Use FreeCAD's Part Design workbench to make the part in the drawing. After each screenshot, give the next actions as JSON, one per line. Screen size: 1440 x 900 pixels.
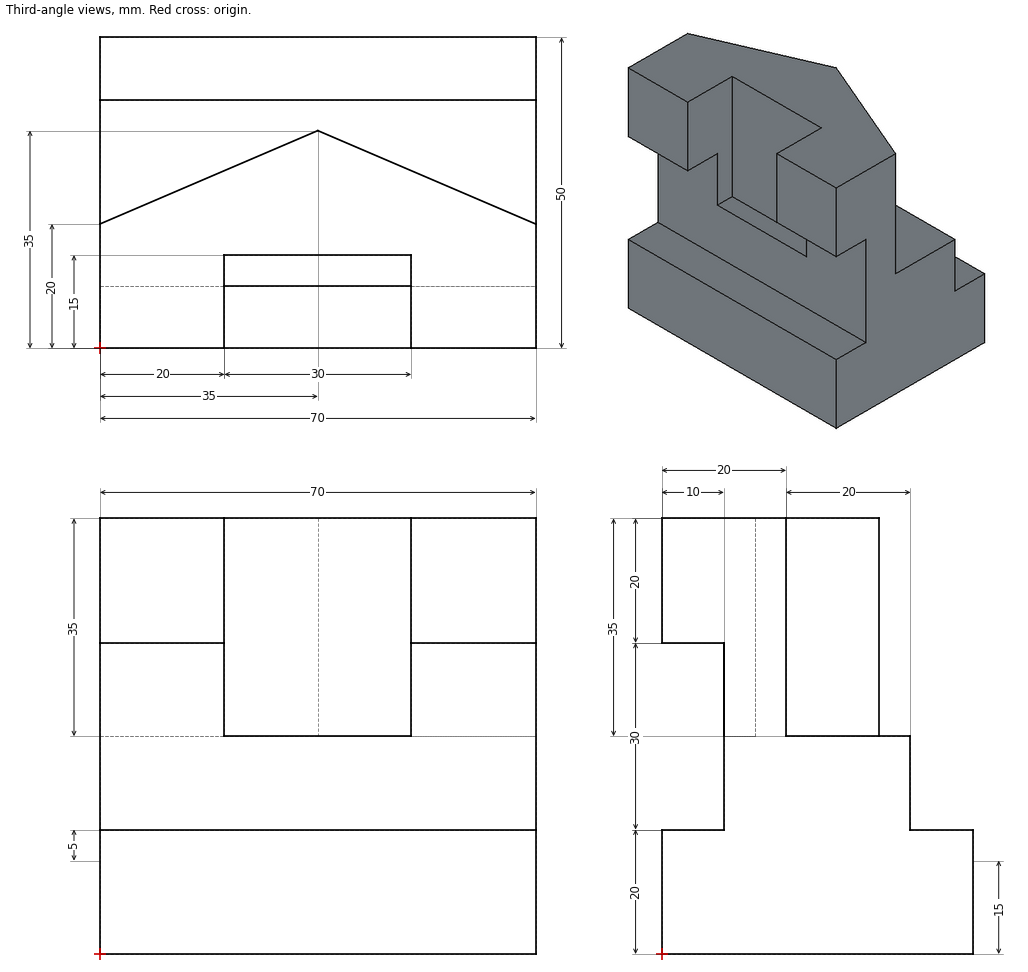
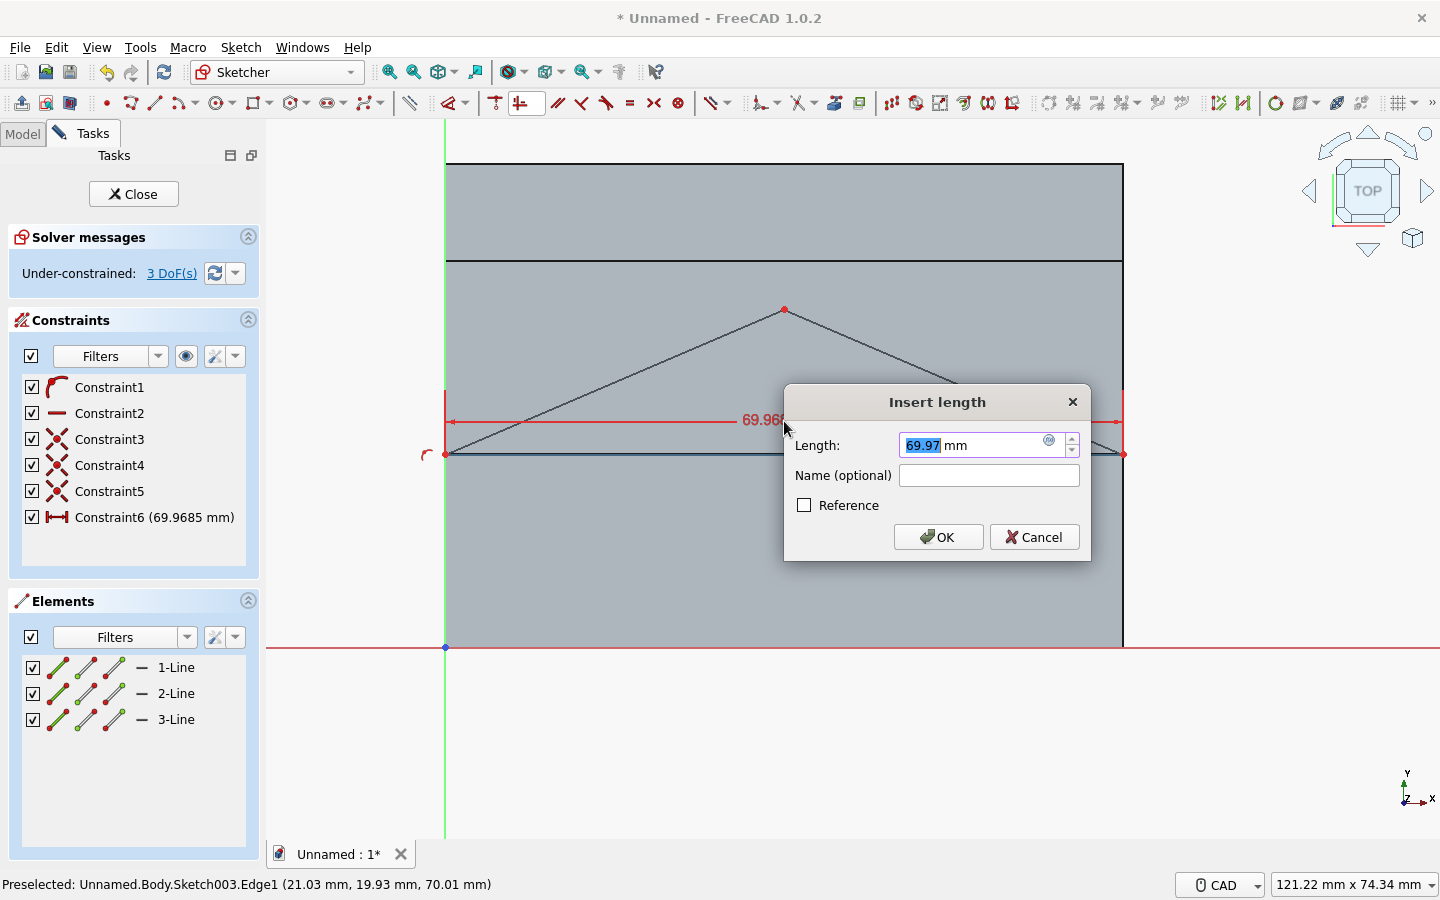
{"action": "type", "text": "70"}
{"action": "key", "text": "Return"}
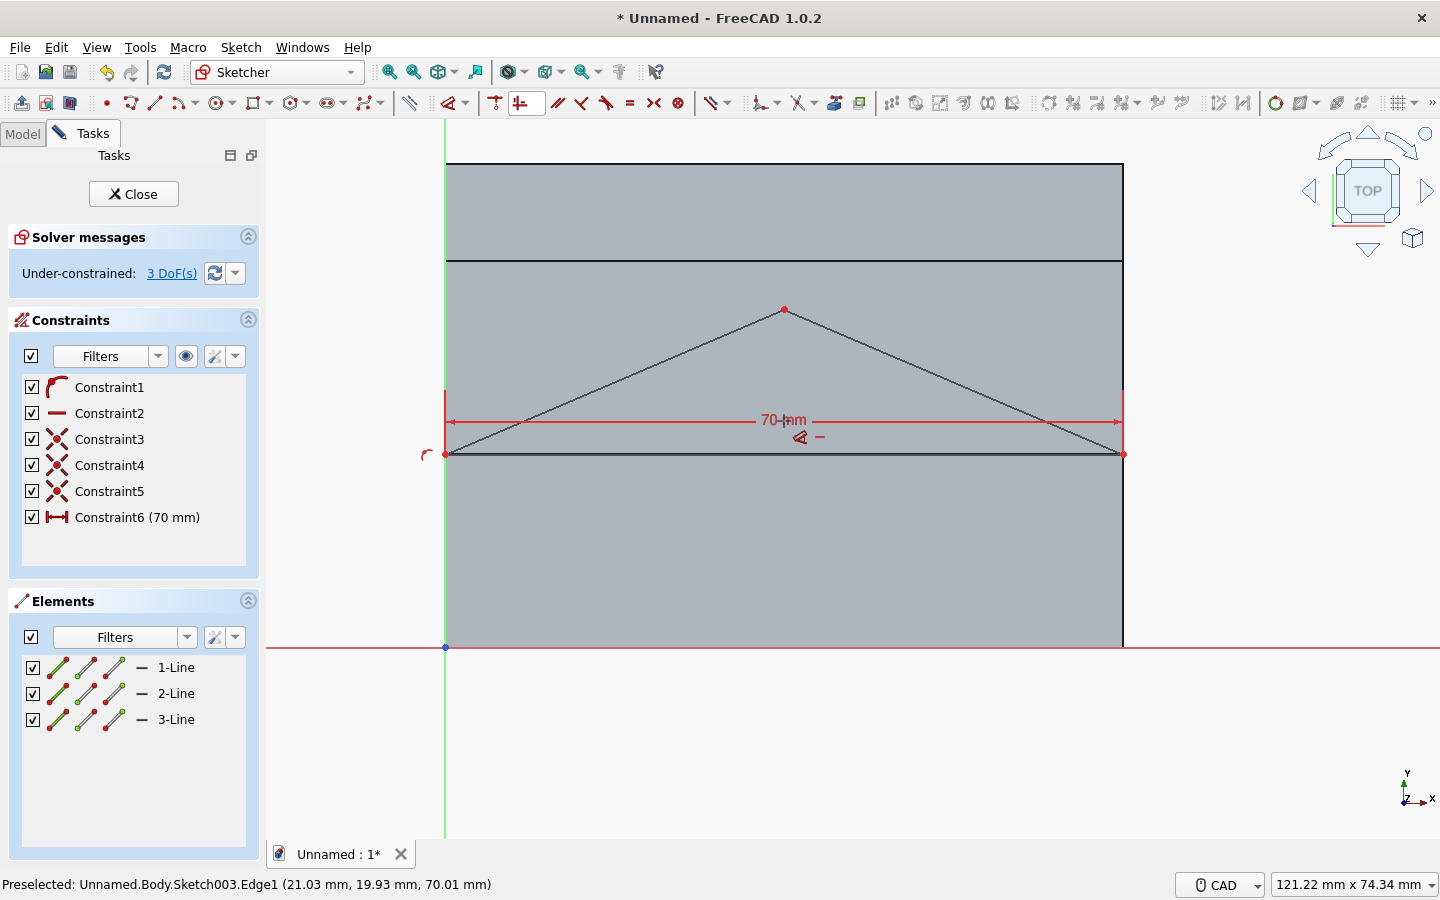
{"action": "left_click", "coordinate": [445, 455]}
{"action": "left_click", "coordinate": [411, 551]}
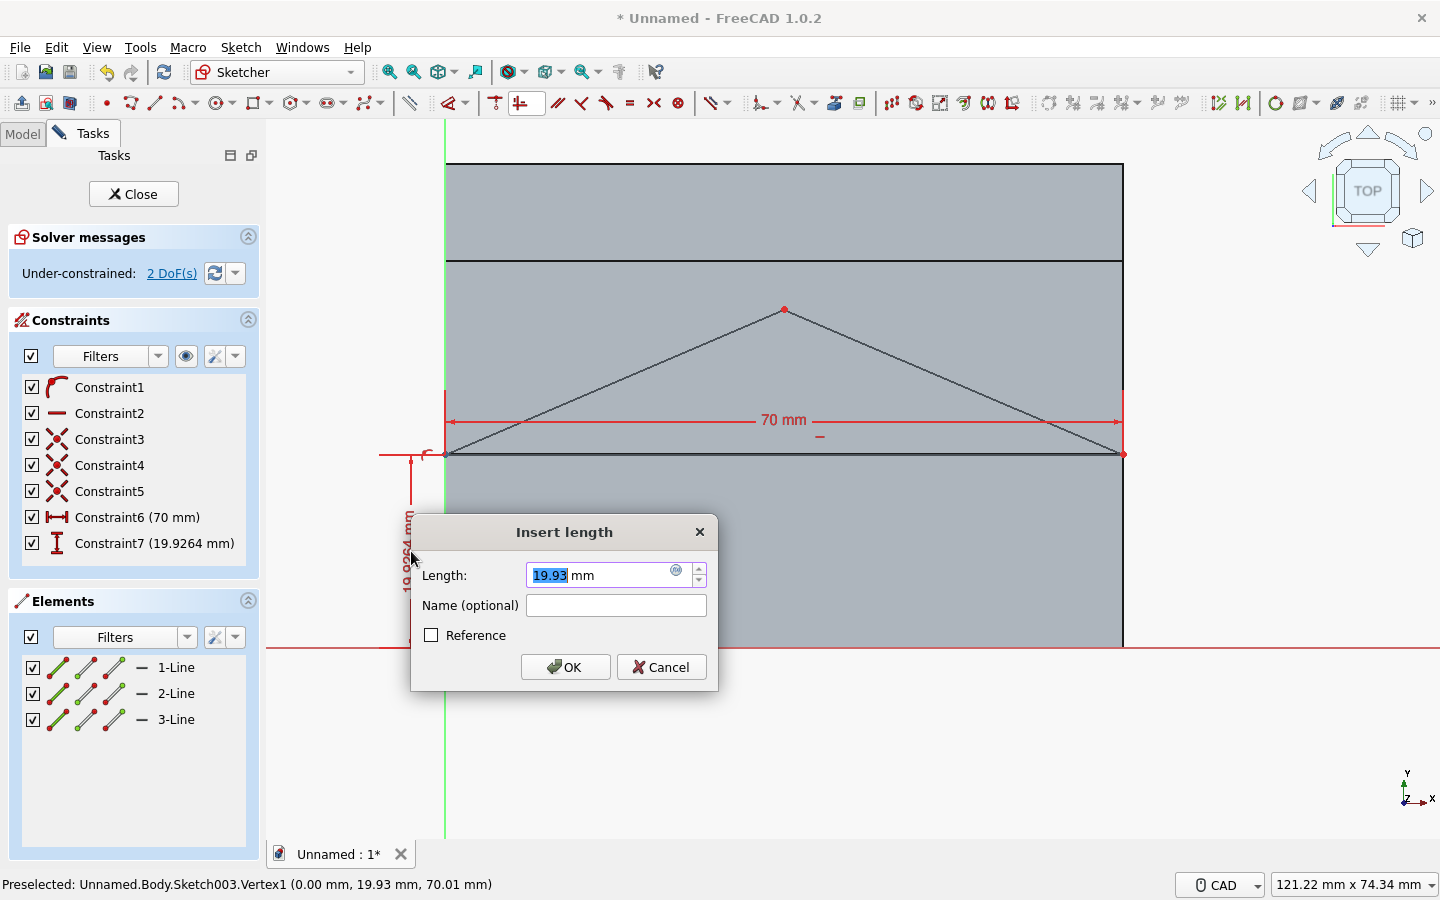
{"action": "type", "text": "20"}
{"action": "key", "text": "Return"}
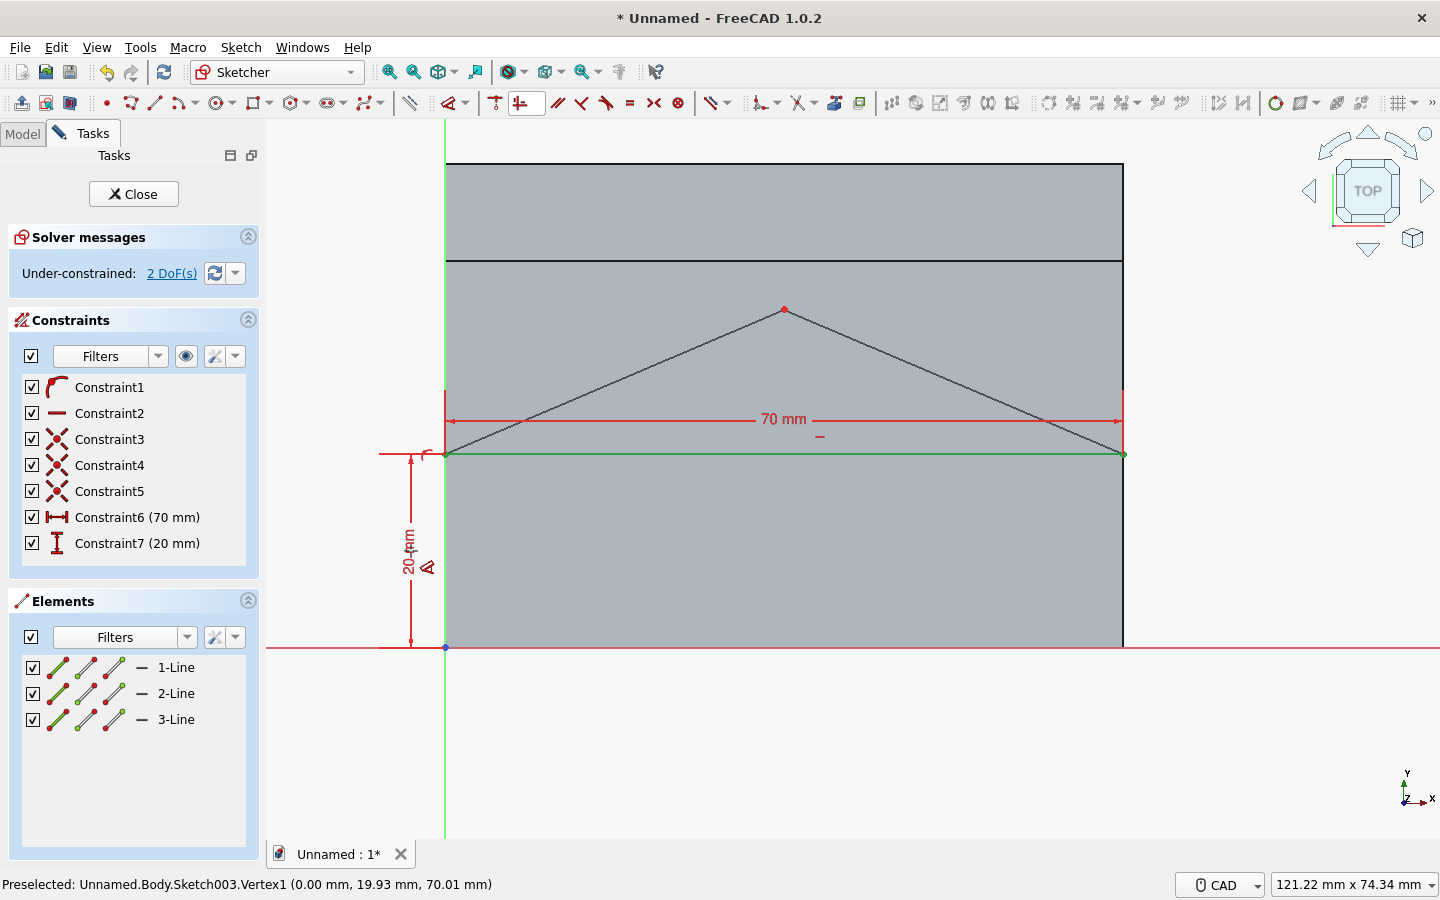
{"action": "left_click", "coordinate": [784, 310]}
{"action": "left_click", "coordinate": [615, 682]}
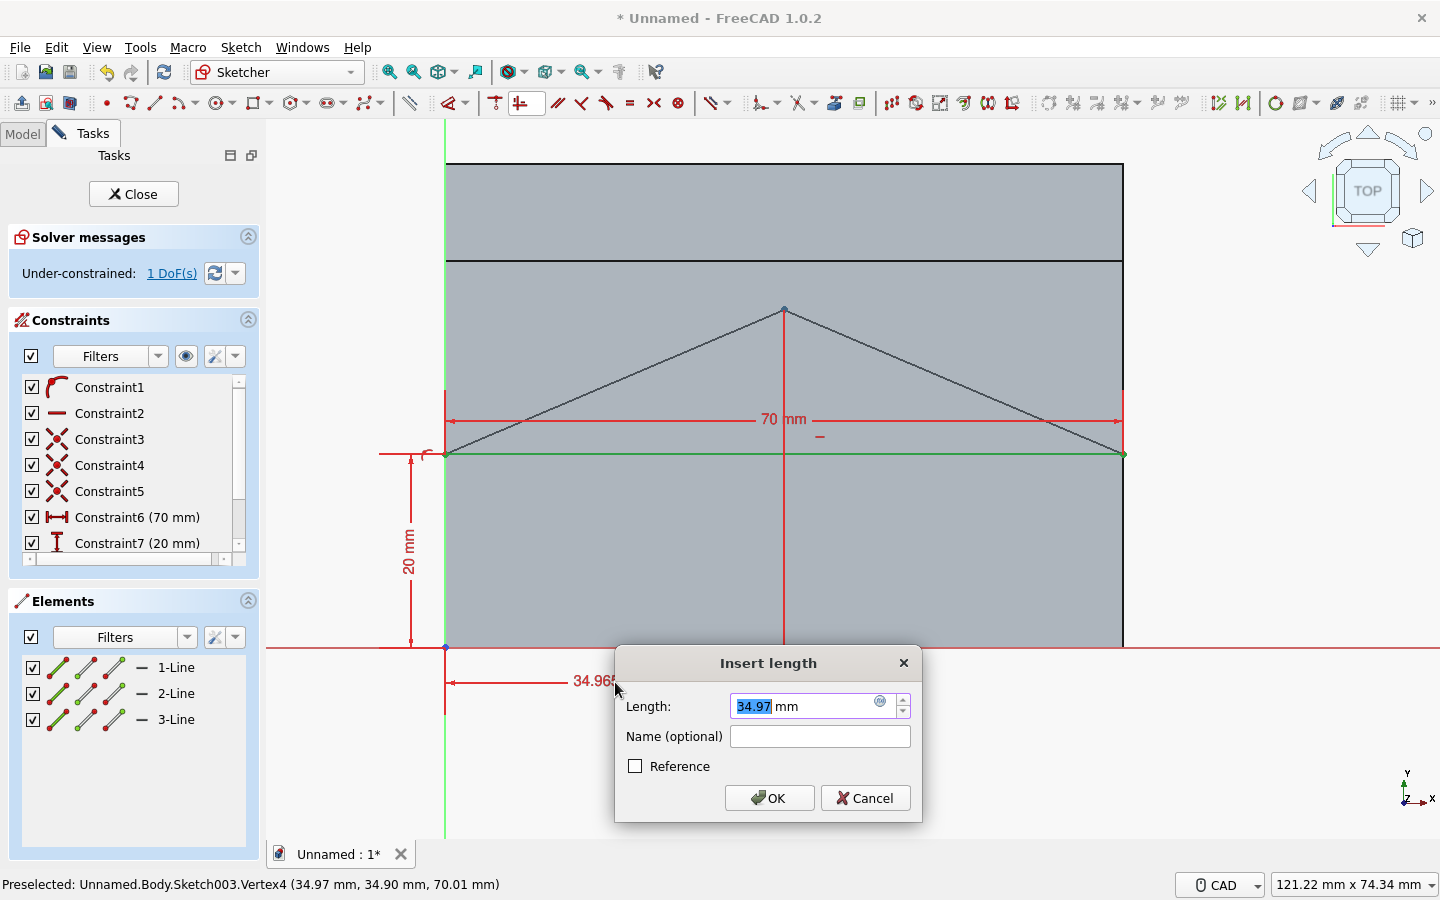
{"action": "type", "text": "35"}
{"action": "key", "text": "Return"}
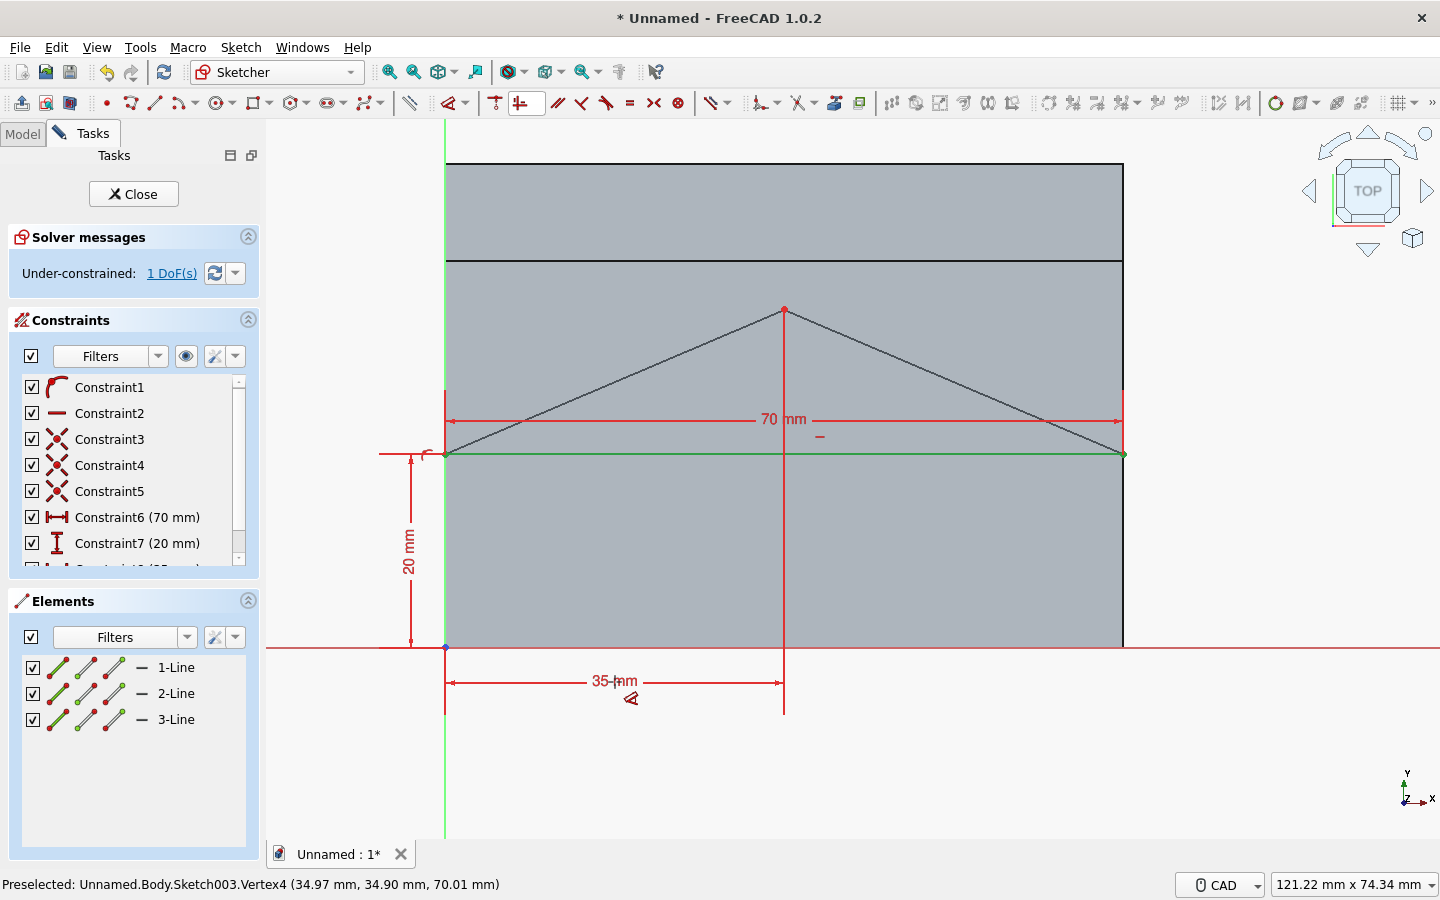
{"action": "left_click", "coordinate": [784, 310]}
{"action": "left_click", "coordinate": [411, 479]}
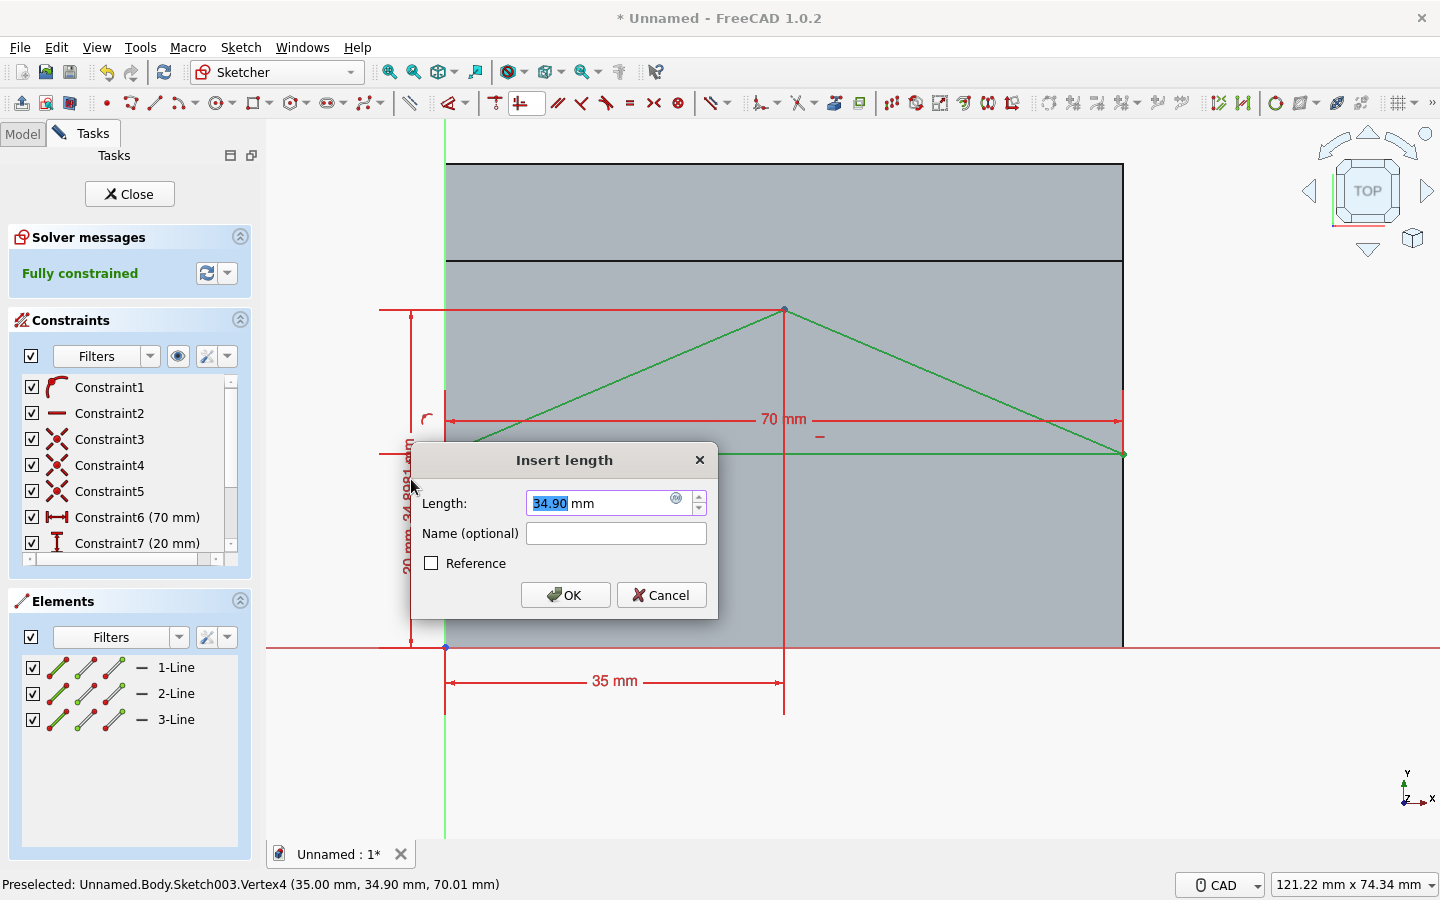
{"action": "type", "text": "35"}
{"action": "key", "text": "Return"}
{"action": "key", "text": "Escape"}